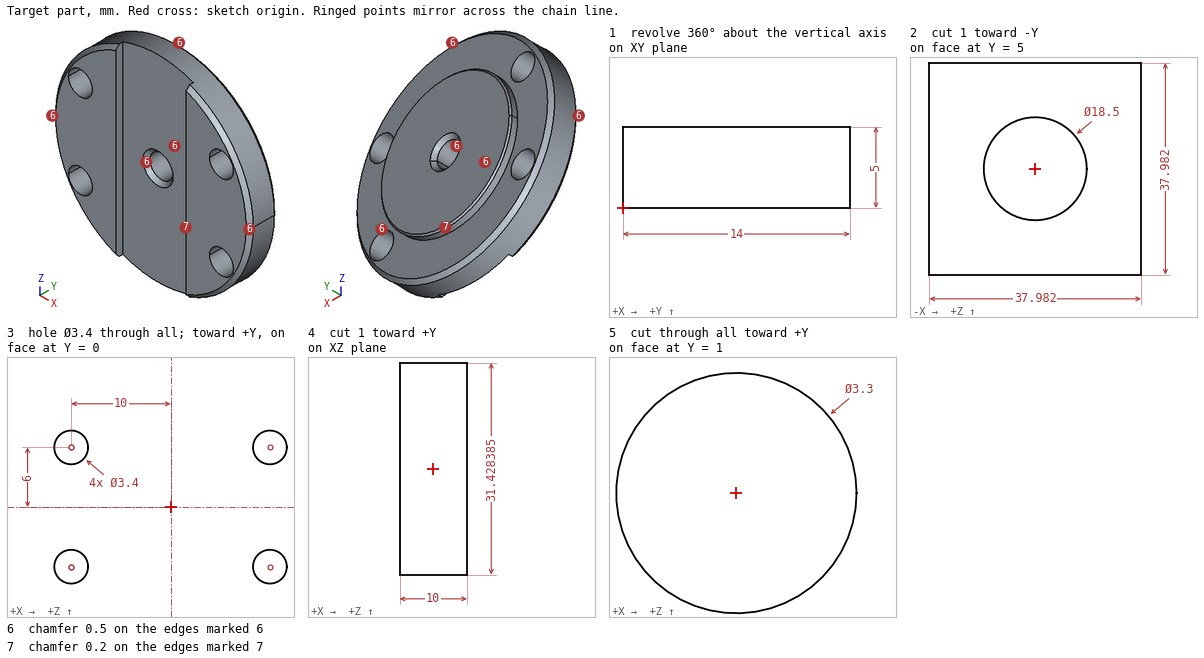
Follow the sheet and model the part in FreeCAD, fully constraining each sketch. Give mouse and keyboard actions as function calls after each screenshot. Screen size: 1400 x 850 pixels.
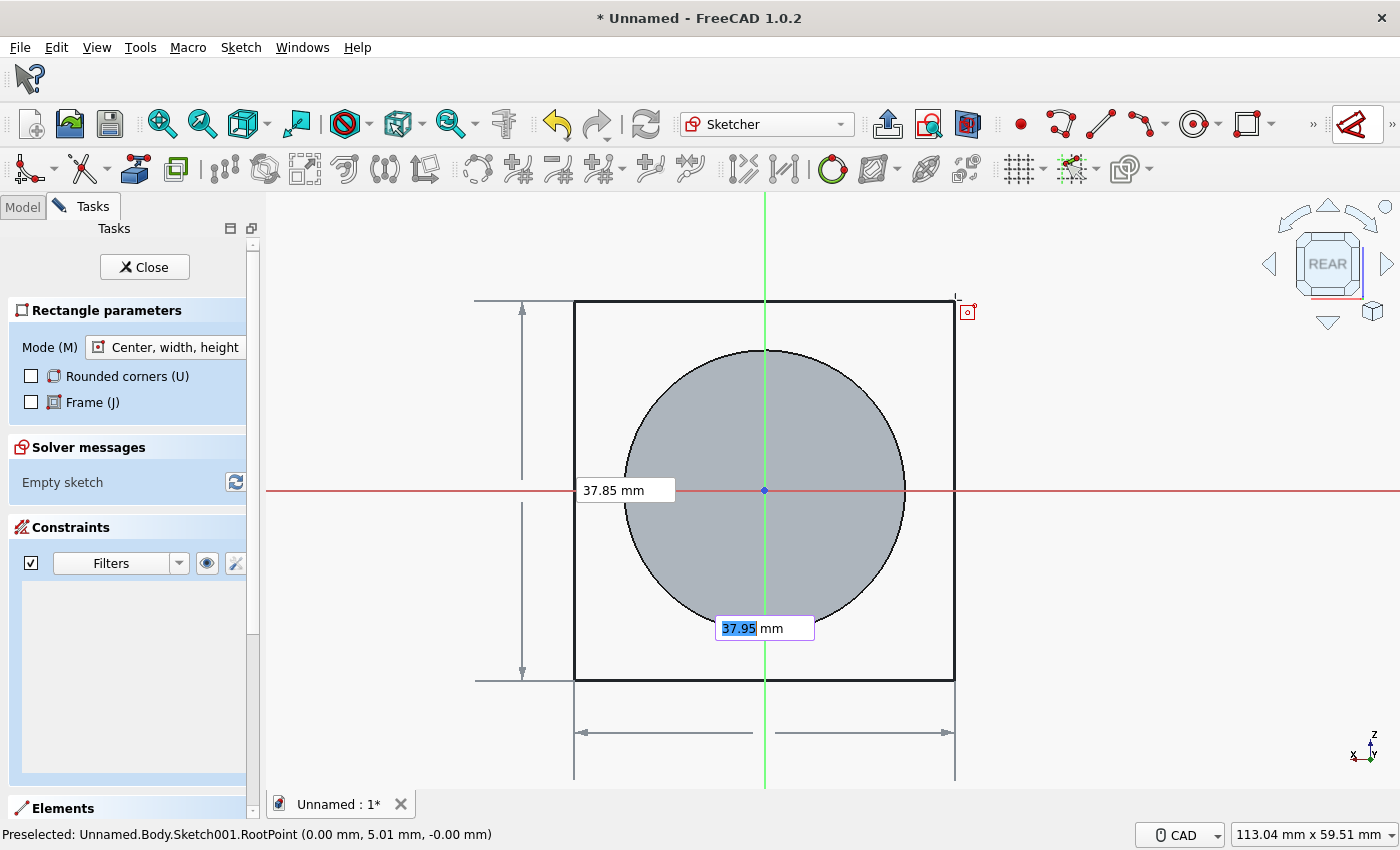
text(37.982)
key(Tab)
text(37.982)
key(Return)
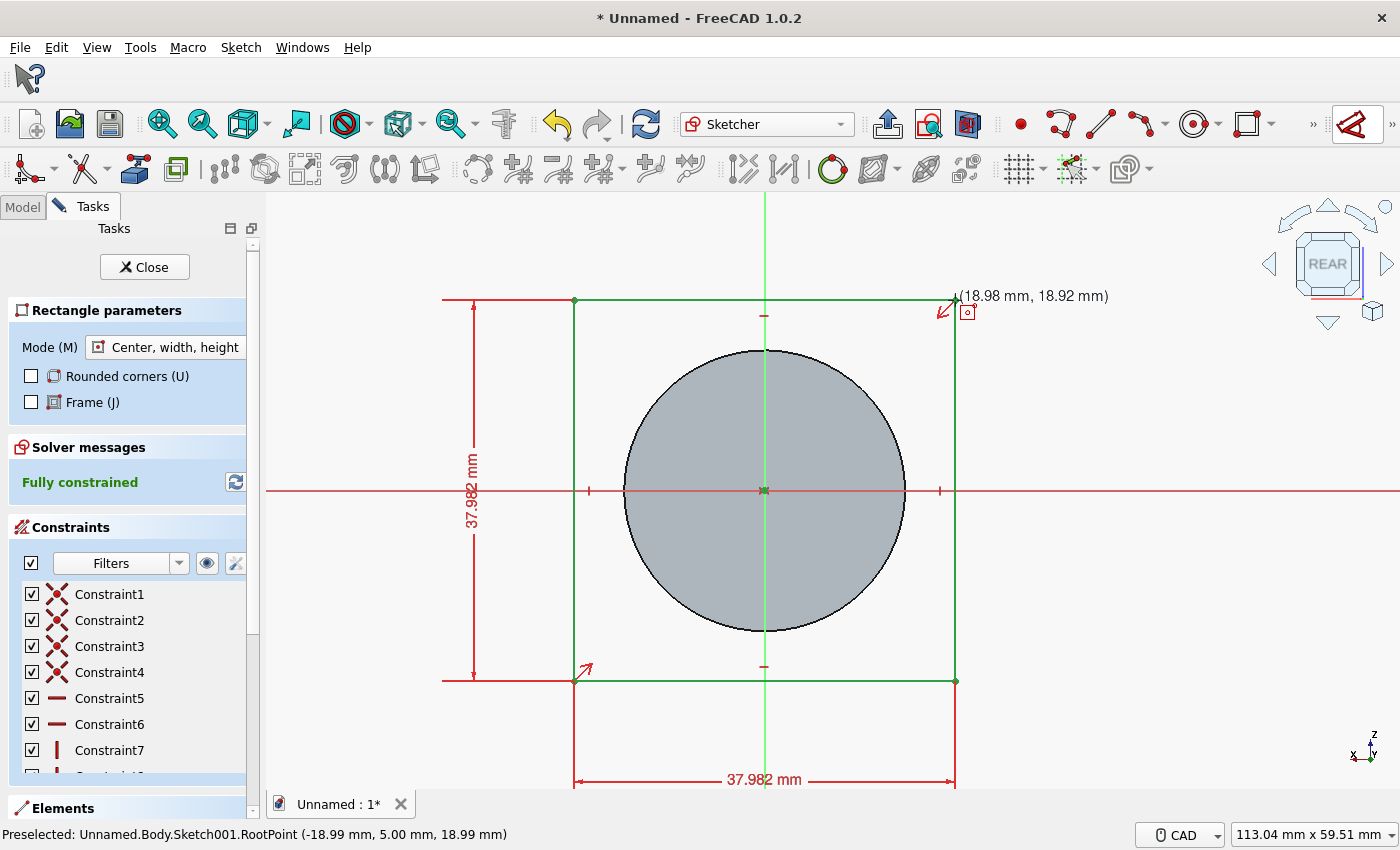
key(g)
key(c)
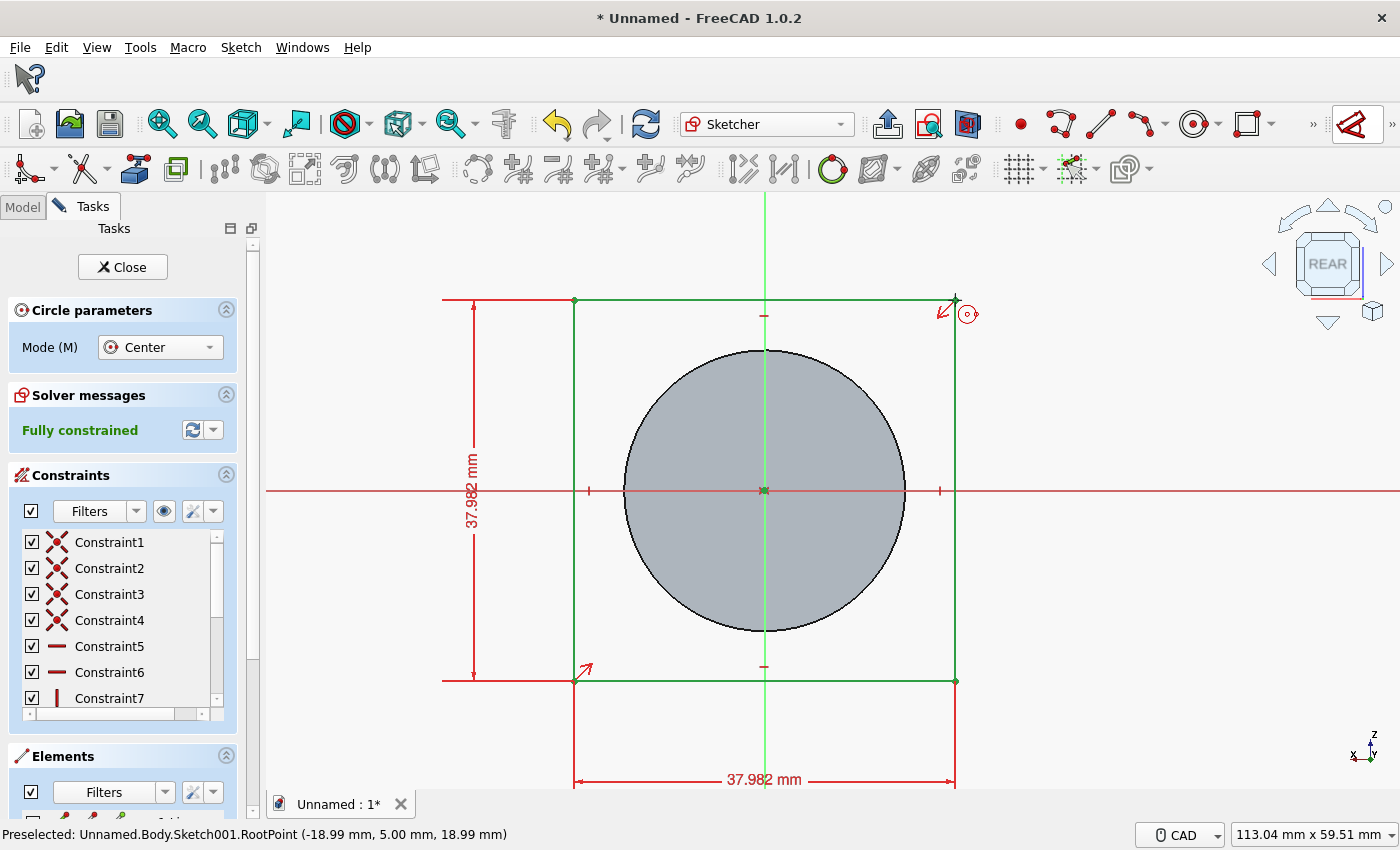
click(765, 491)
move(830, 425)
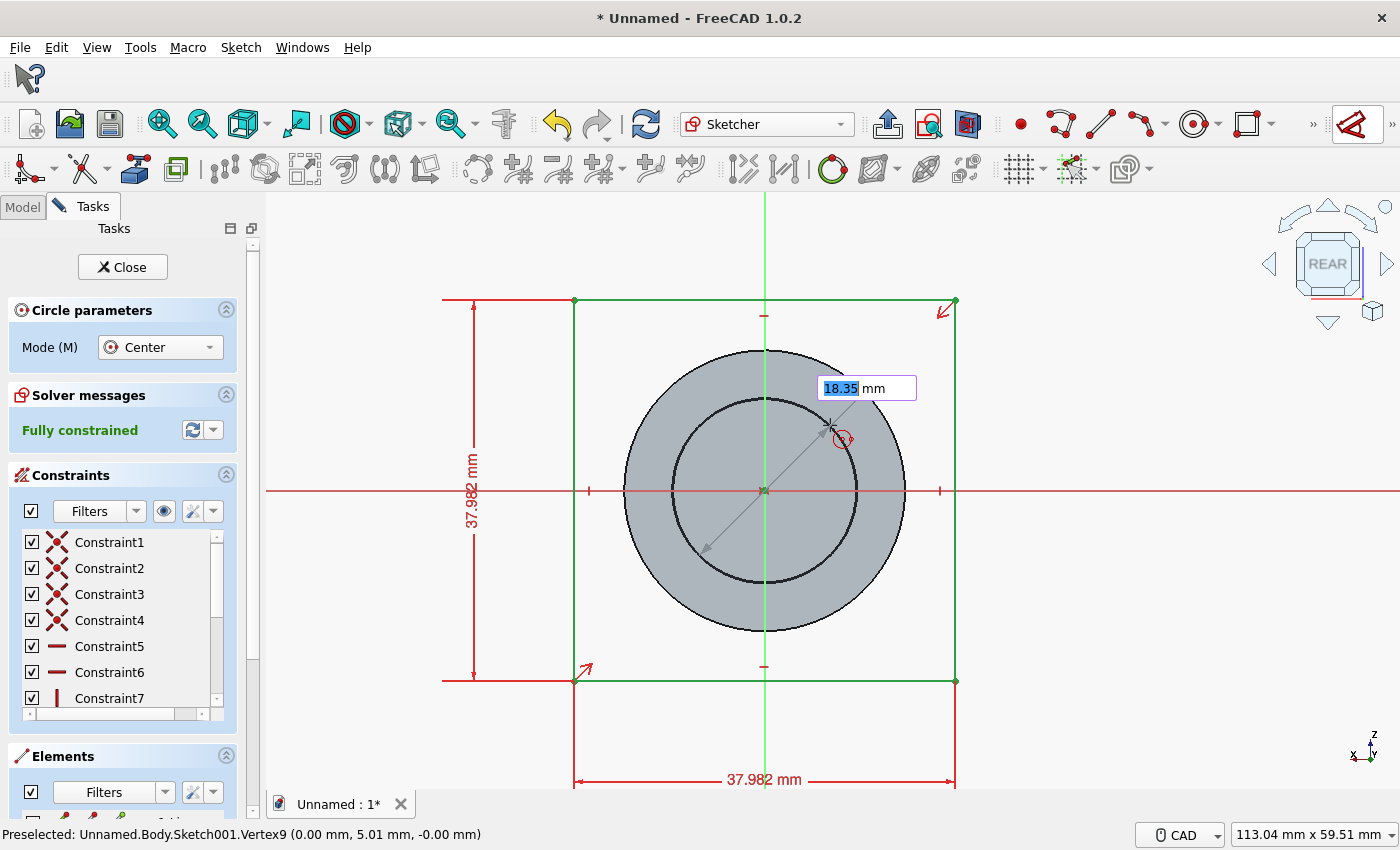
text(18.5)
key(Return)
key(Escape)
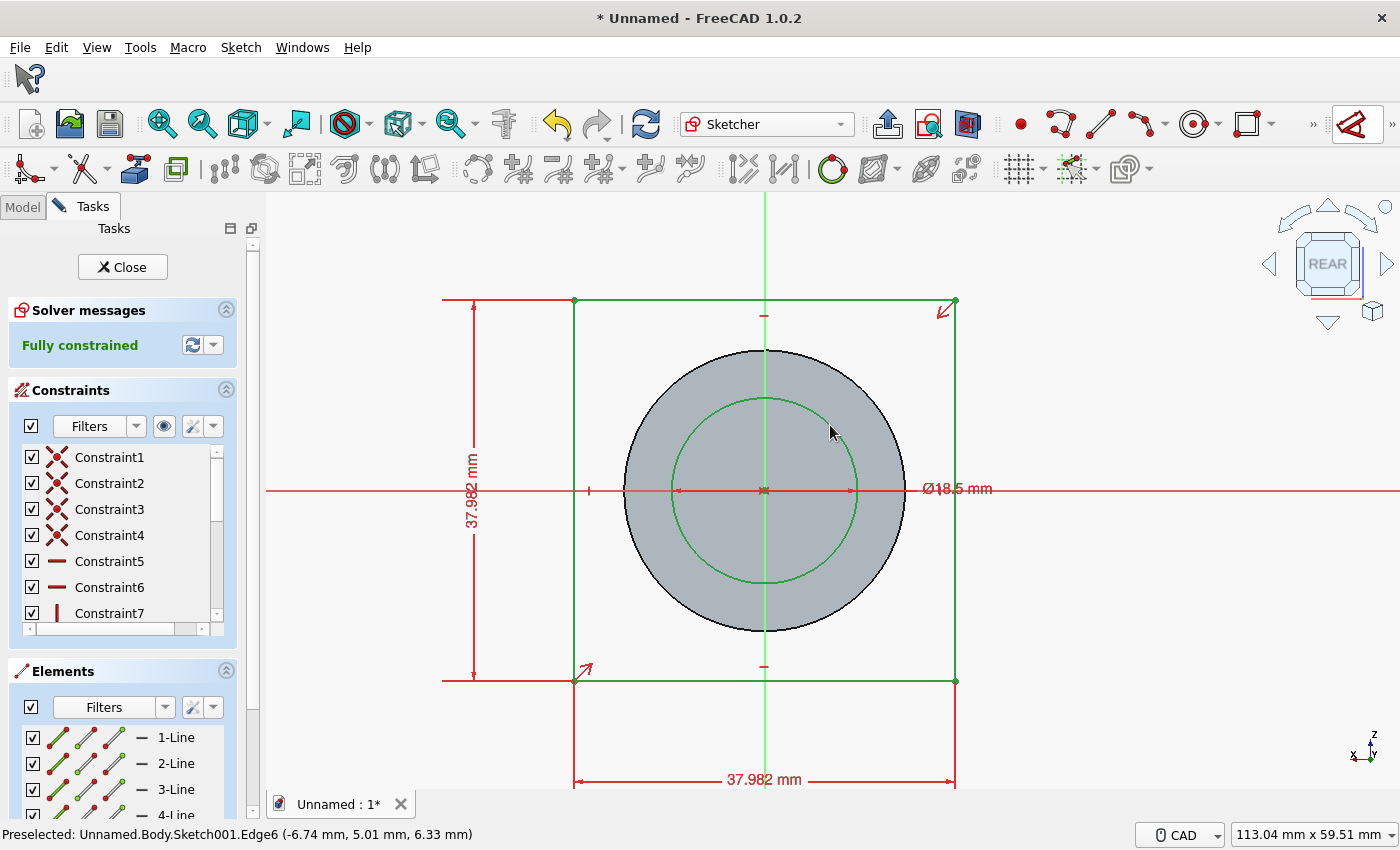
click(123, 267)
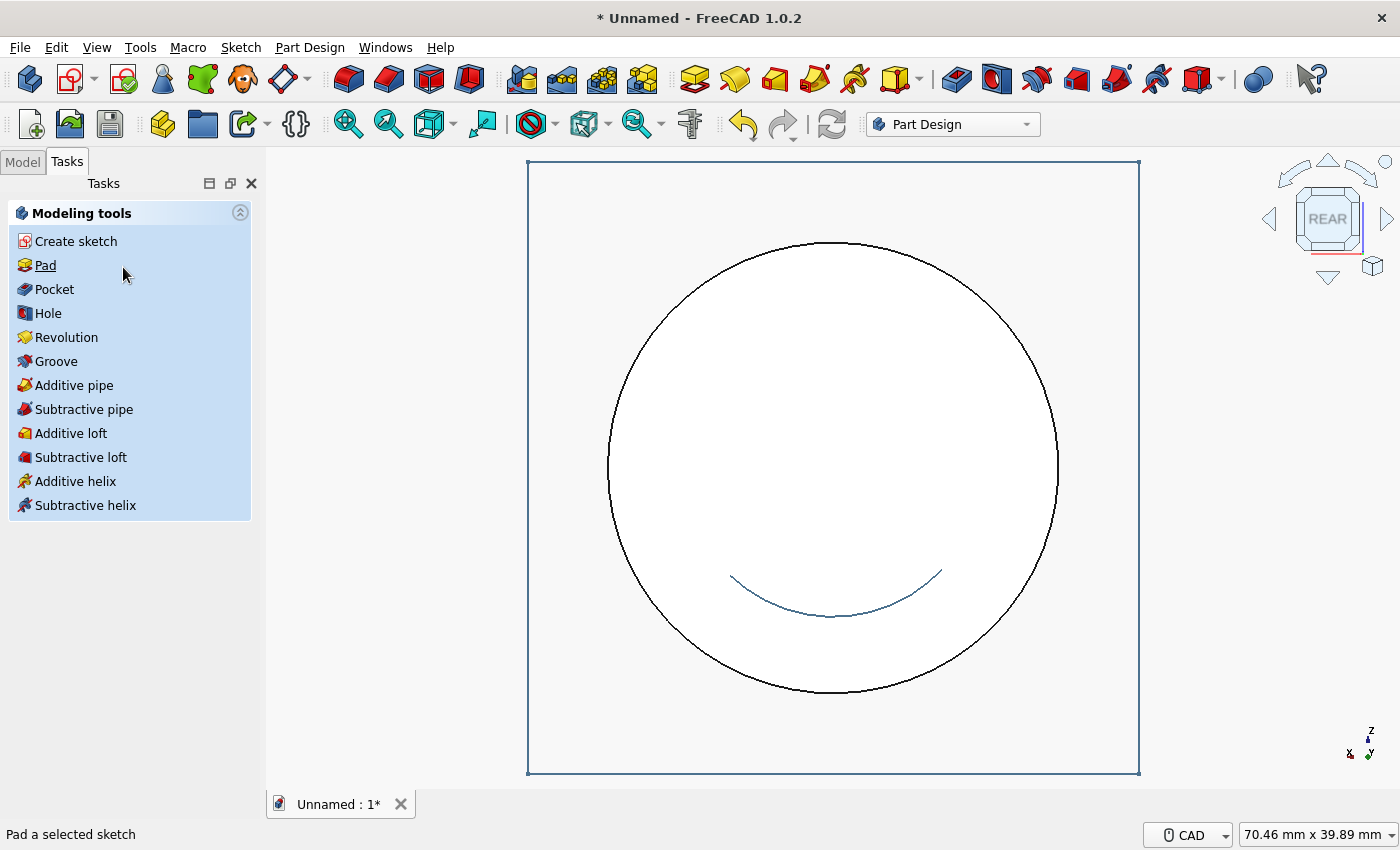
click(958, 80)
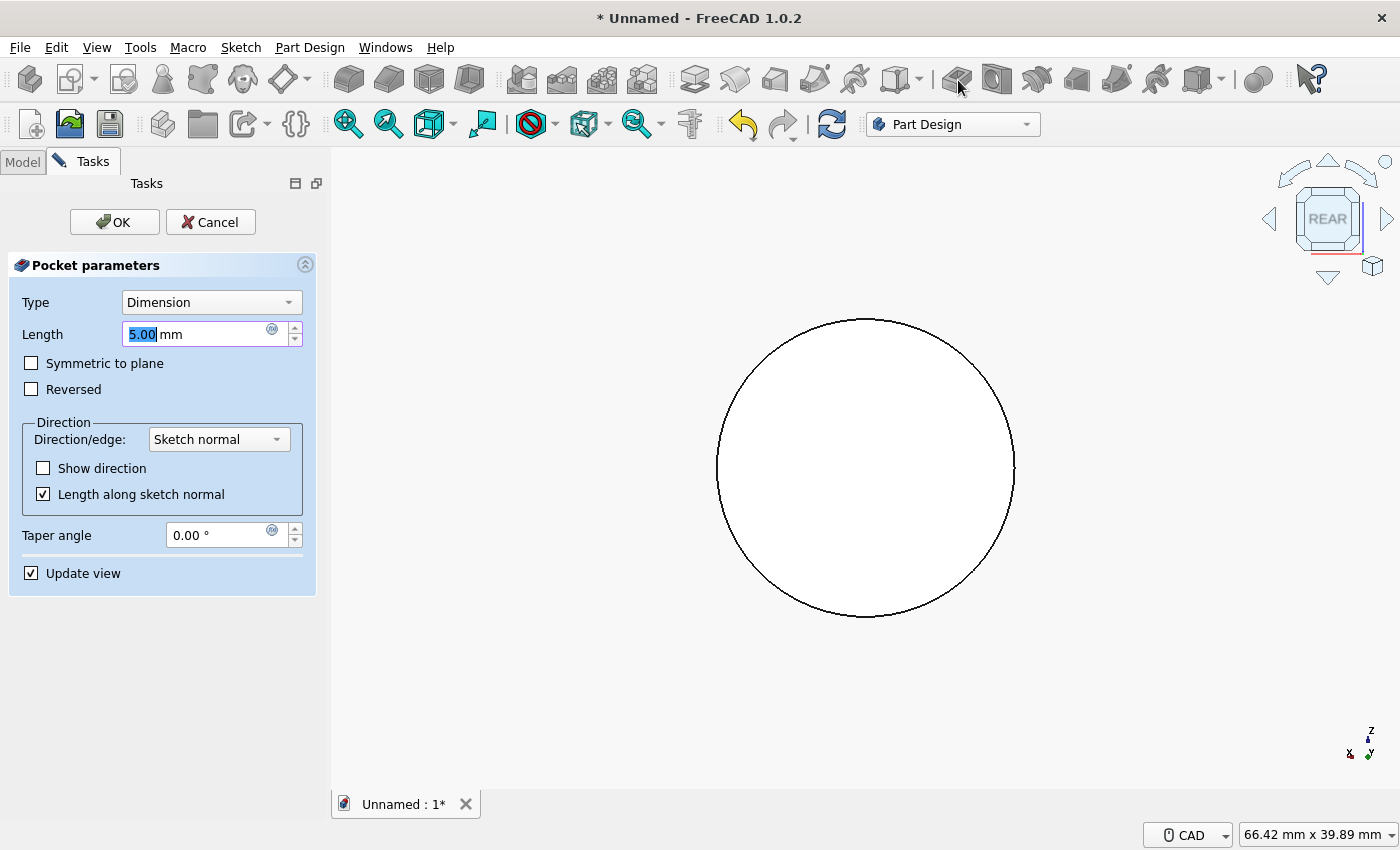
text(1)
key(Tab)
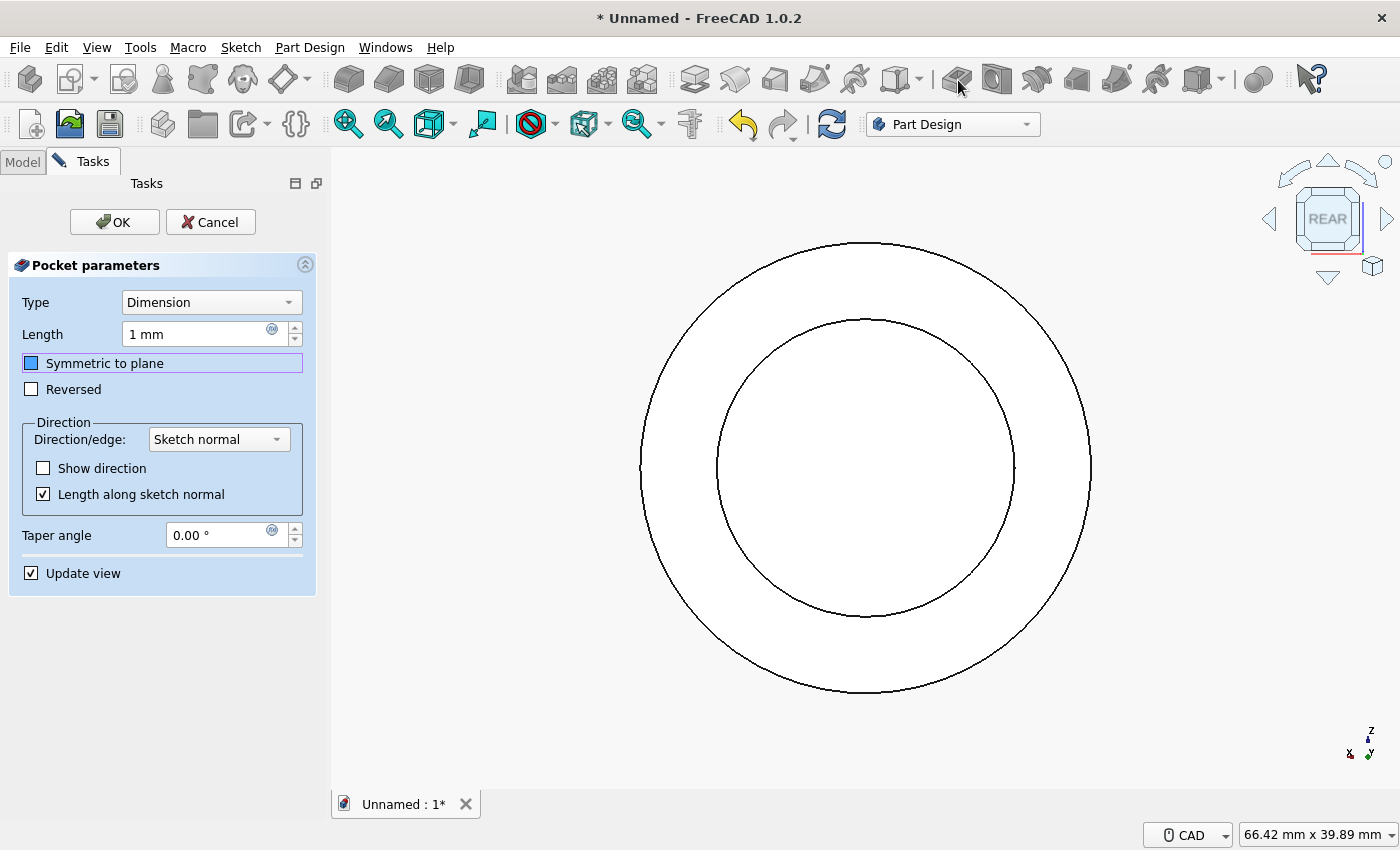
click(115, 222)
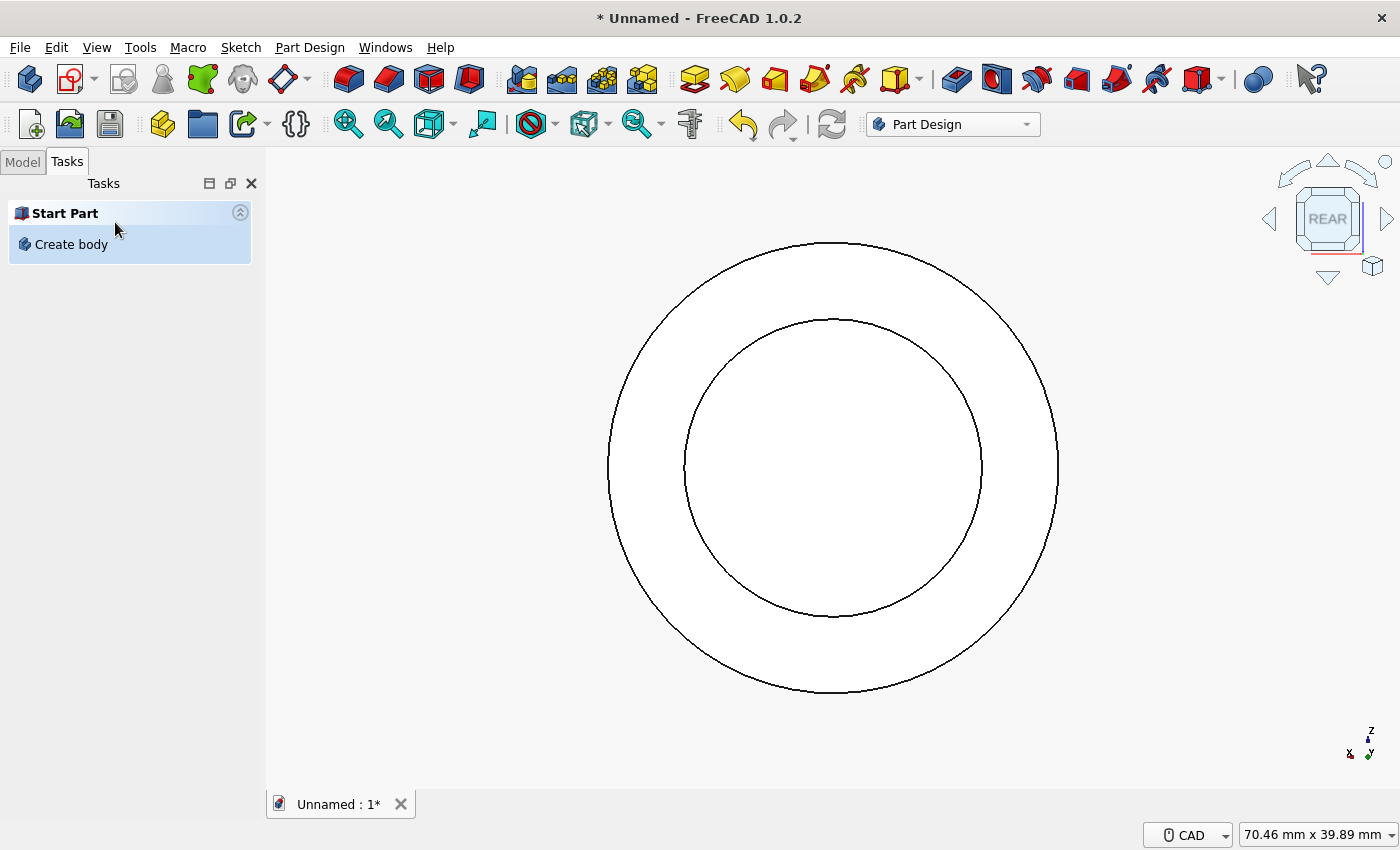
key(0)